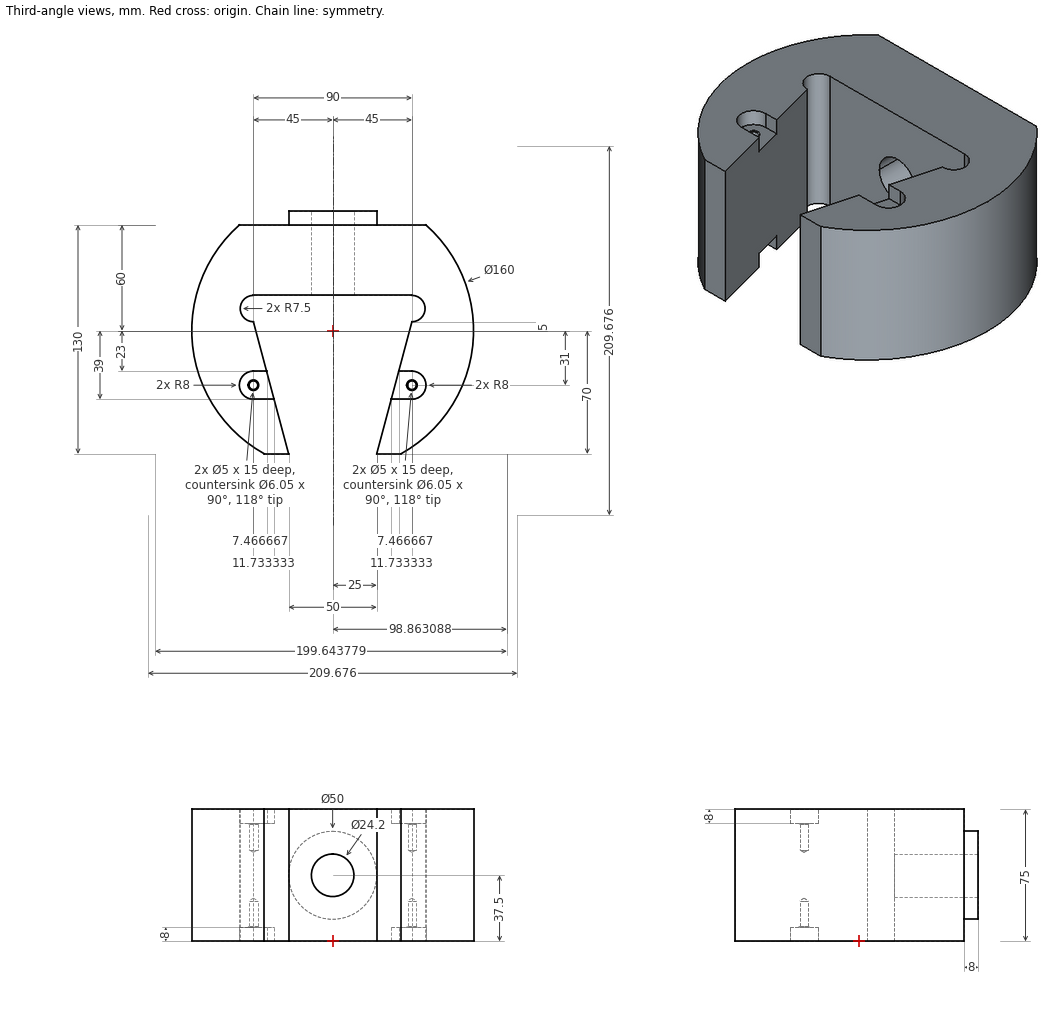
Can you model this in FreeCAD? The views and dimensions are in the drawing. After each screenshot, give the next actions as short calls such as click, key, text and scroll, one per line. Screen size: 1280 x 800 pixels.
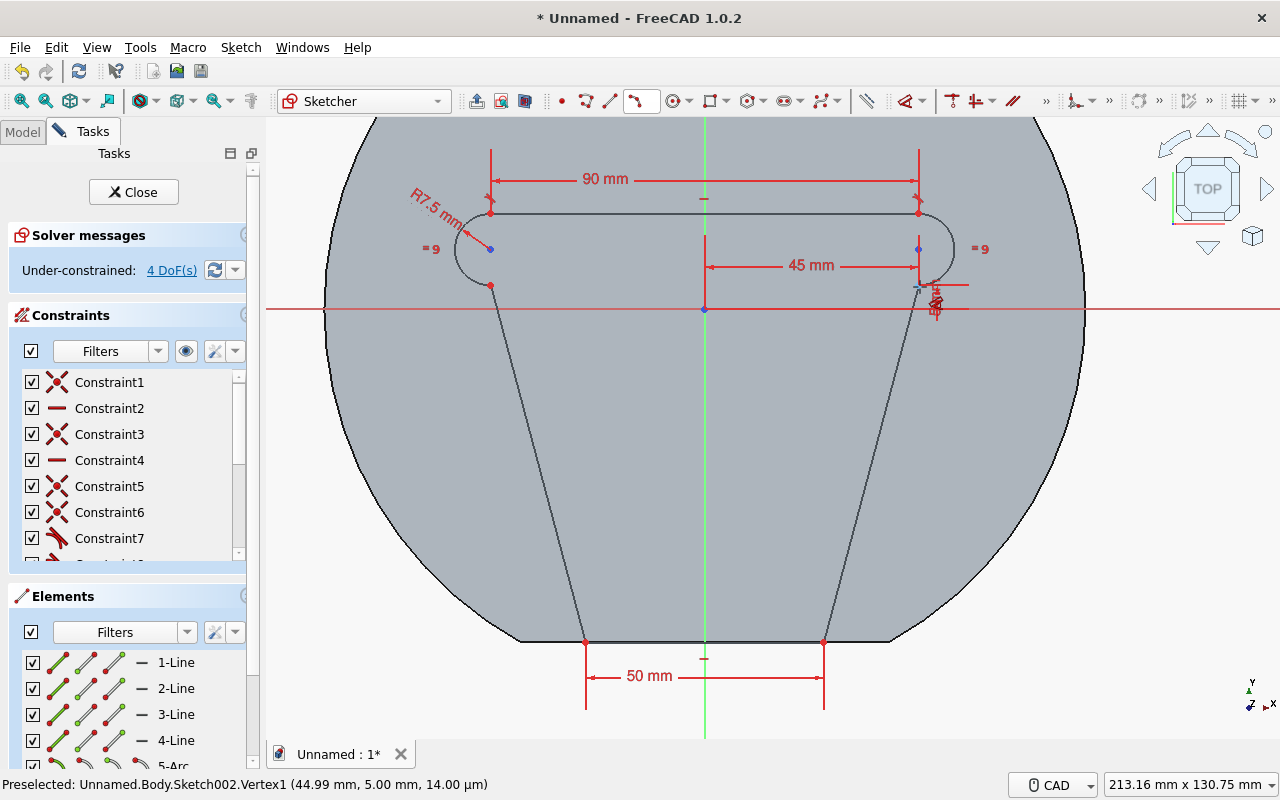
click(824, 643)
click(764, 677)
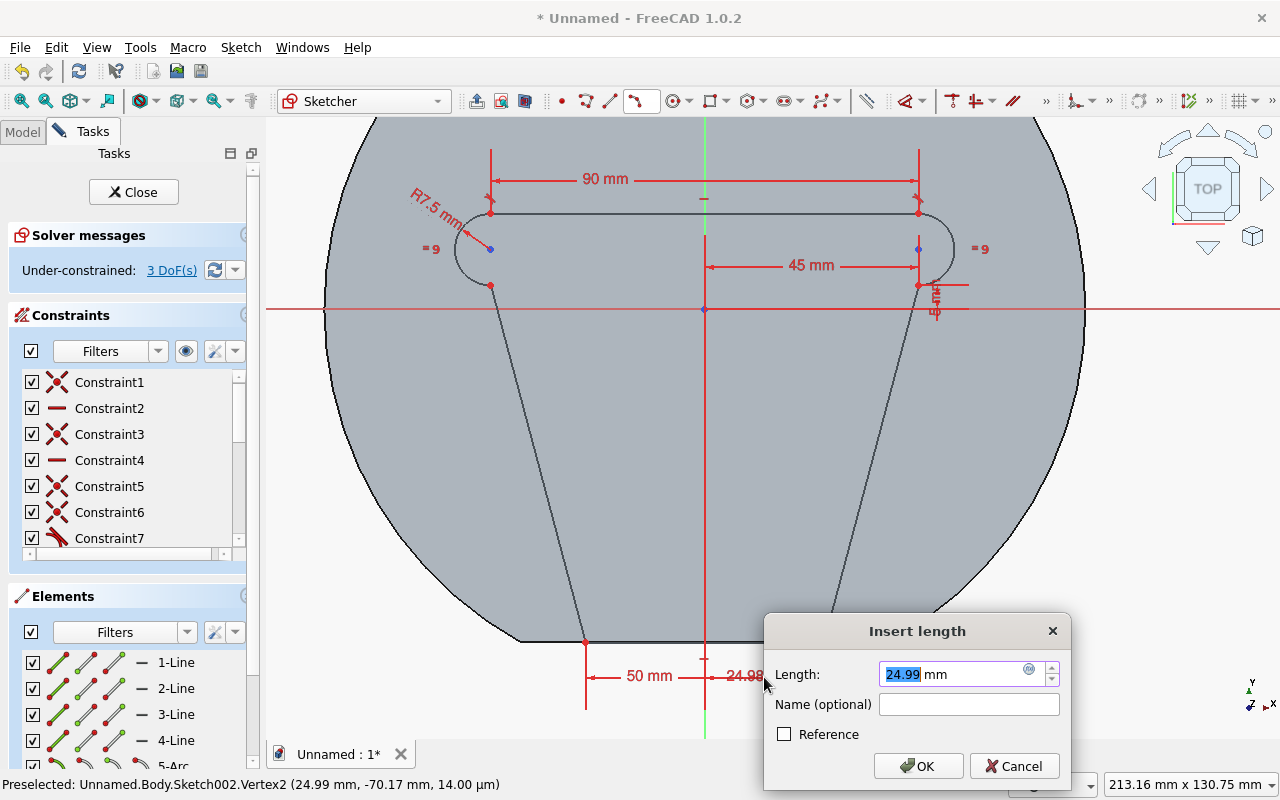
text(25)
key(Return)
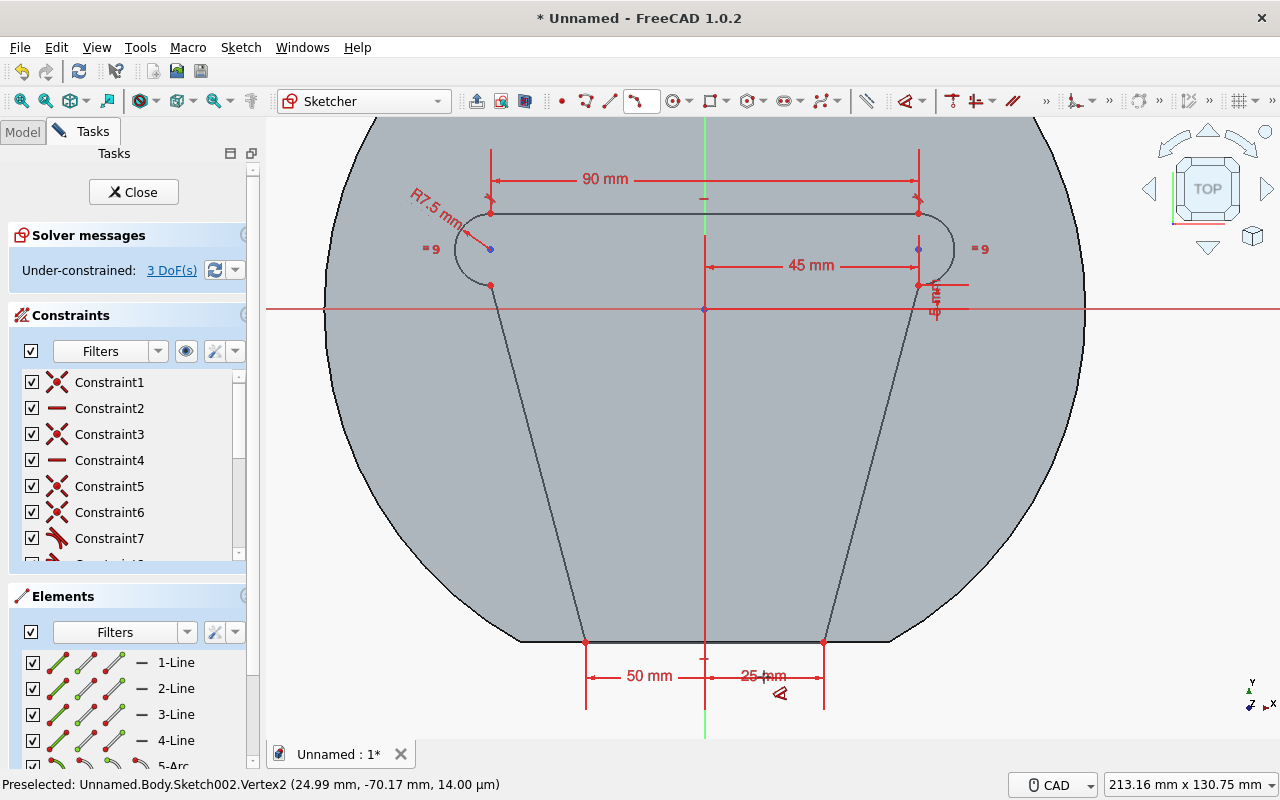
click(824, 643)
click(858, 399)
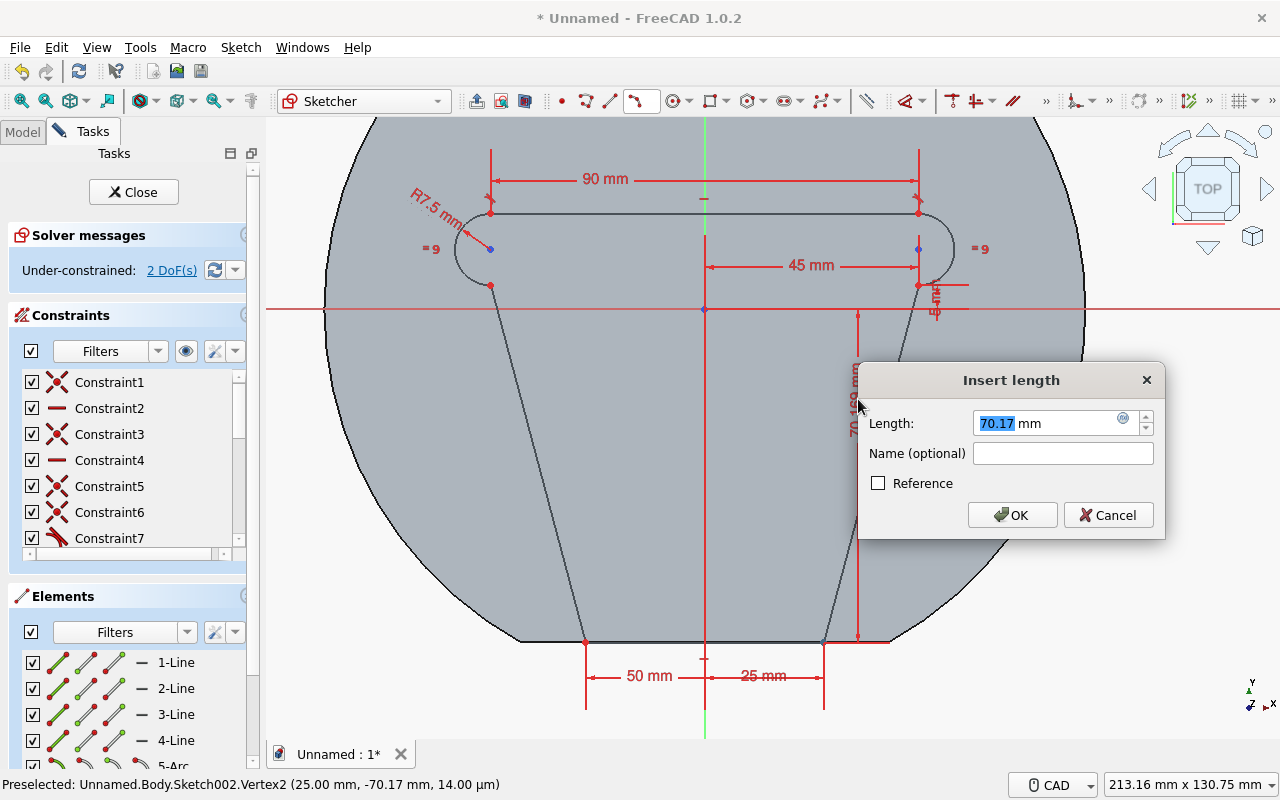
text(70)
key(Return)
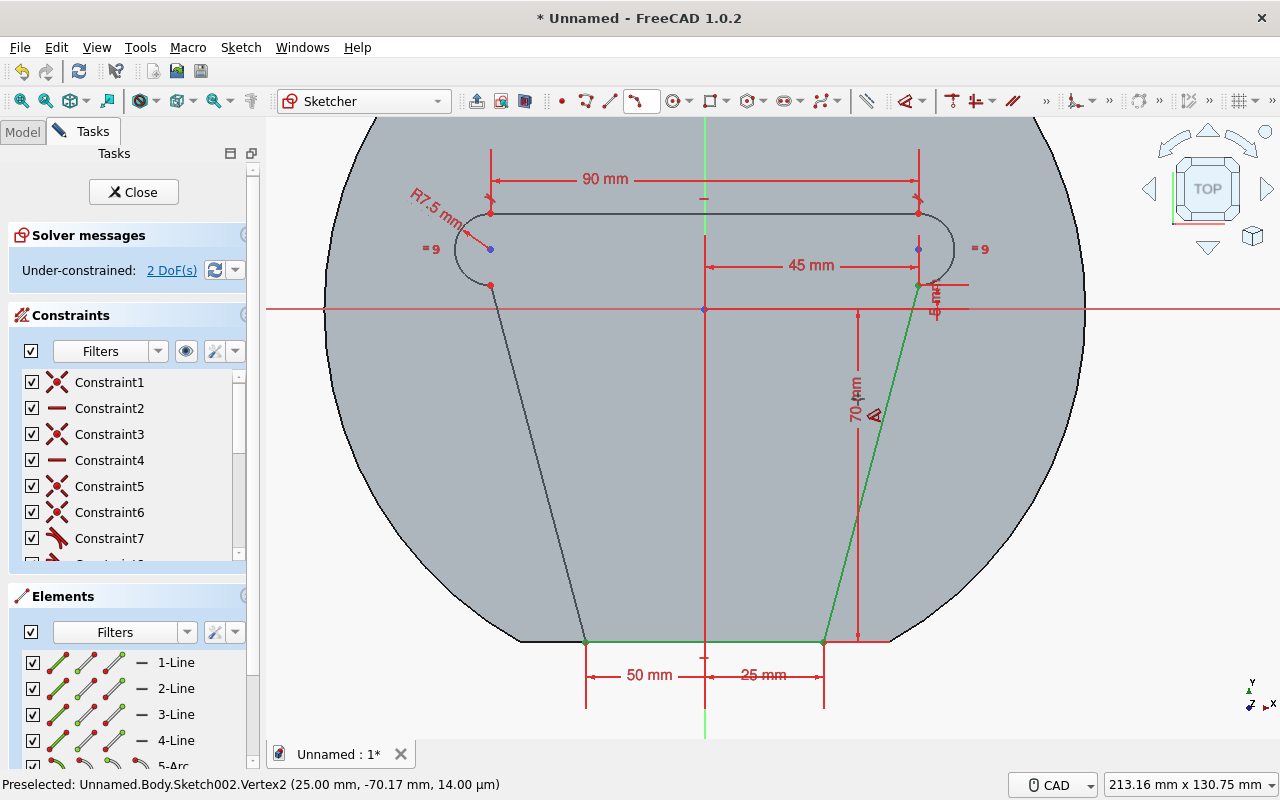
click(491, 285)
click(598, 251)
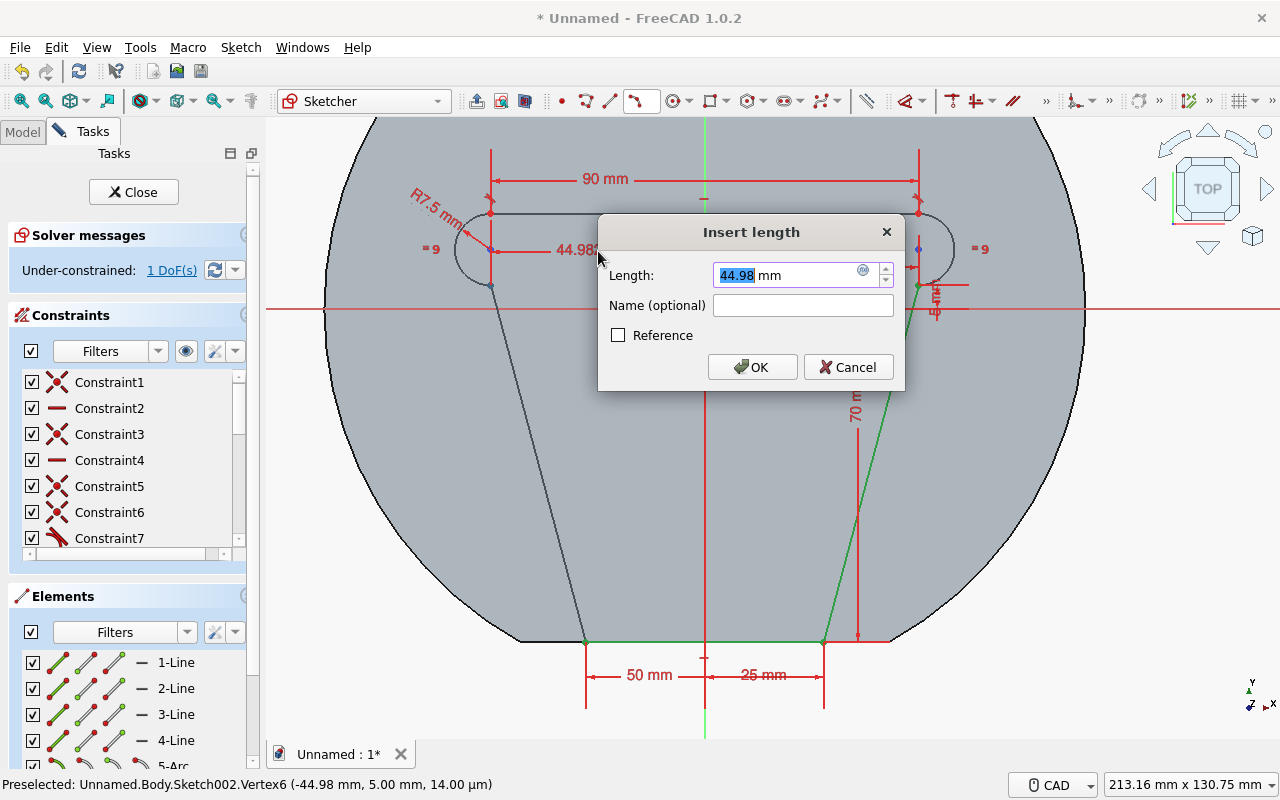
text(45)
key(Return)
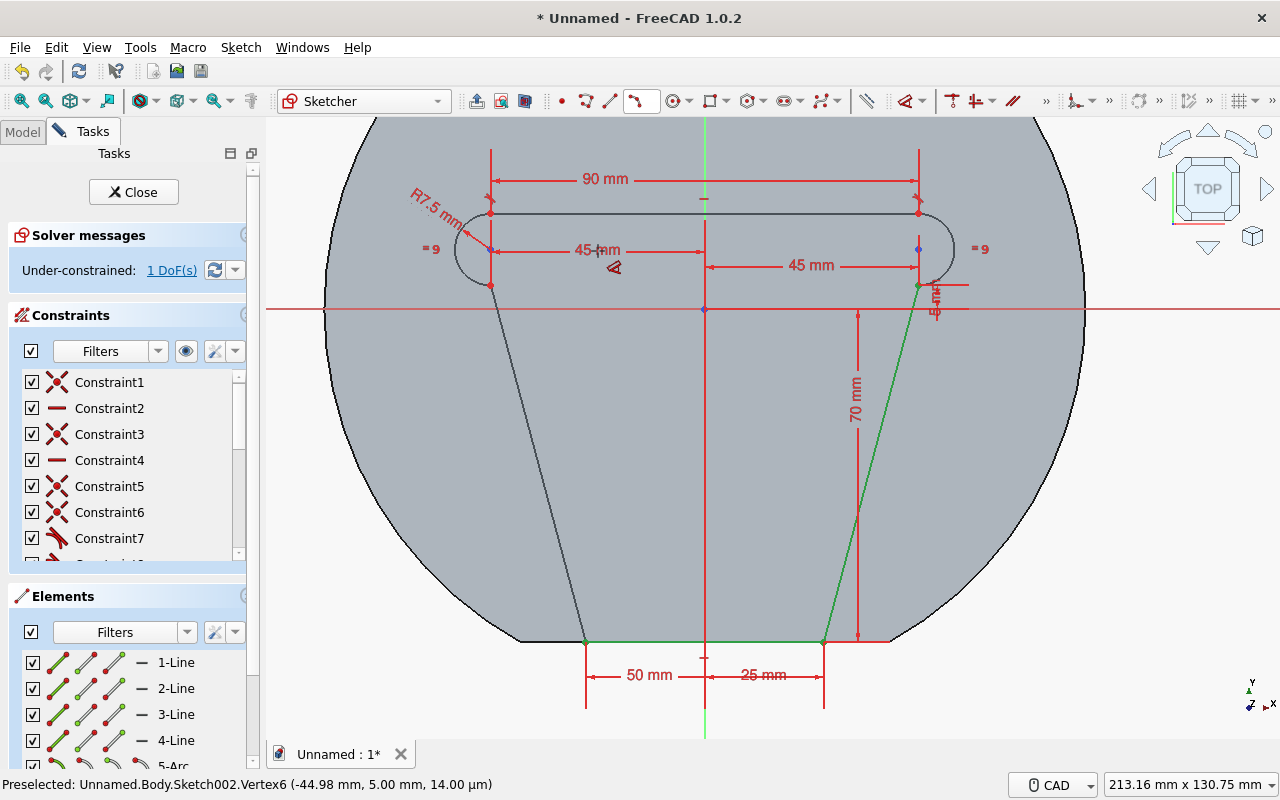
click(491, 214)
click(523, 180)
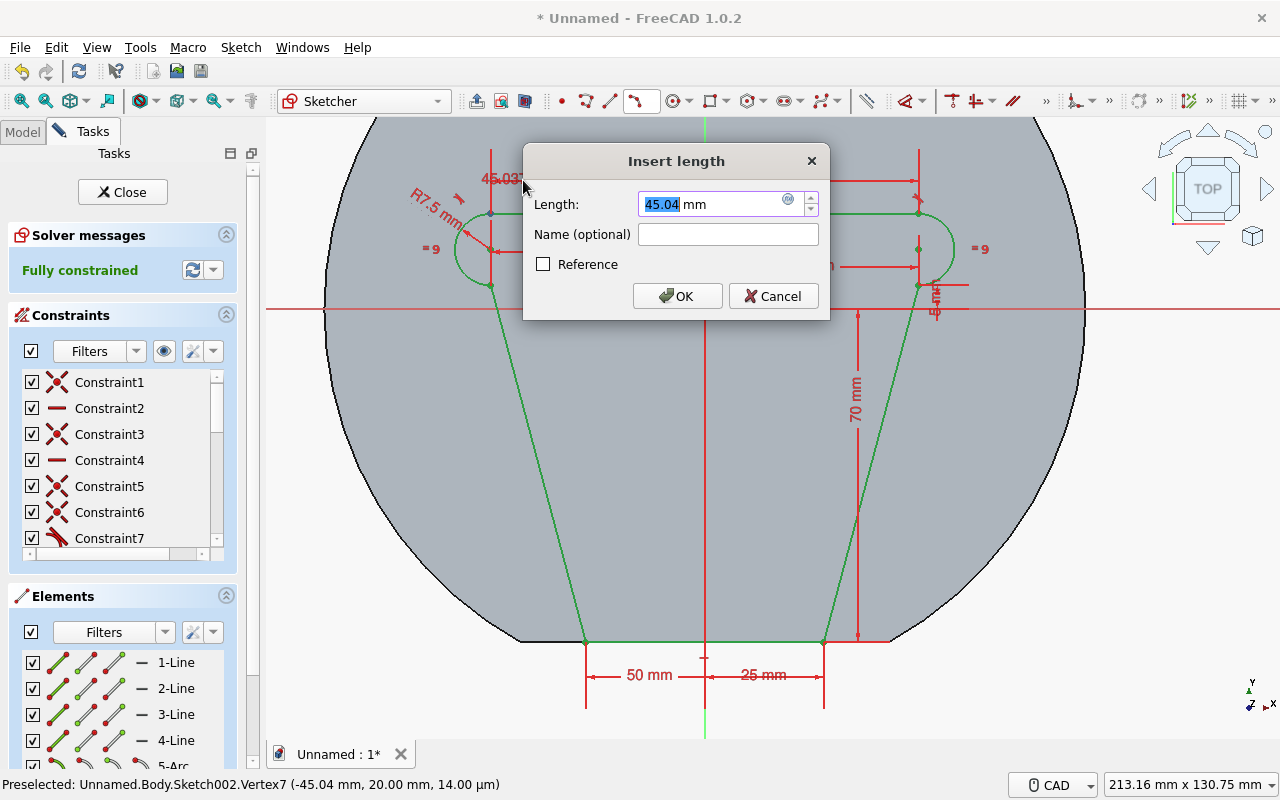
text(45)
key(Return)
key(Escape)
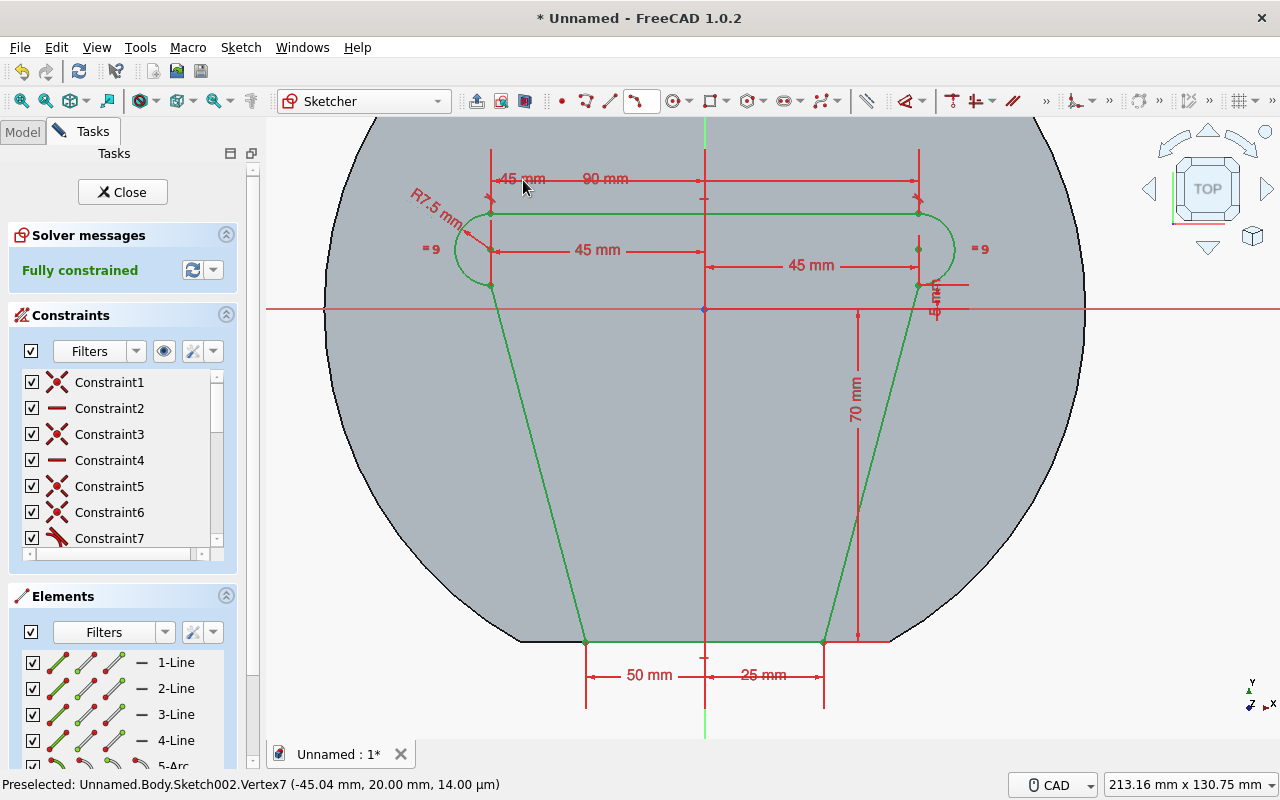
click(123, 192)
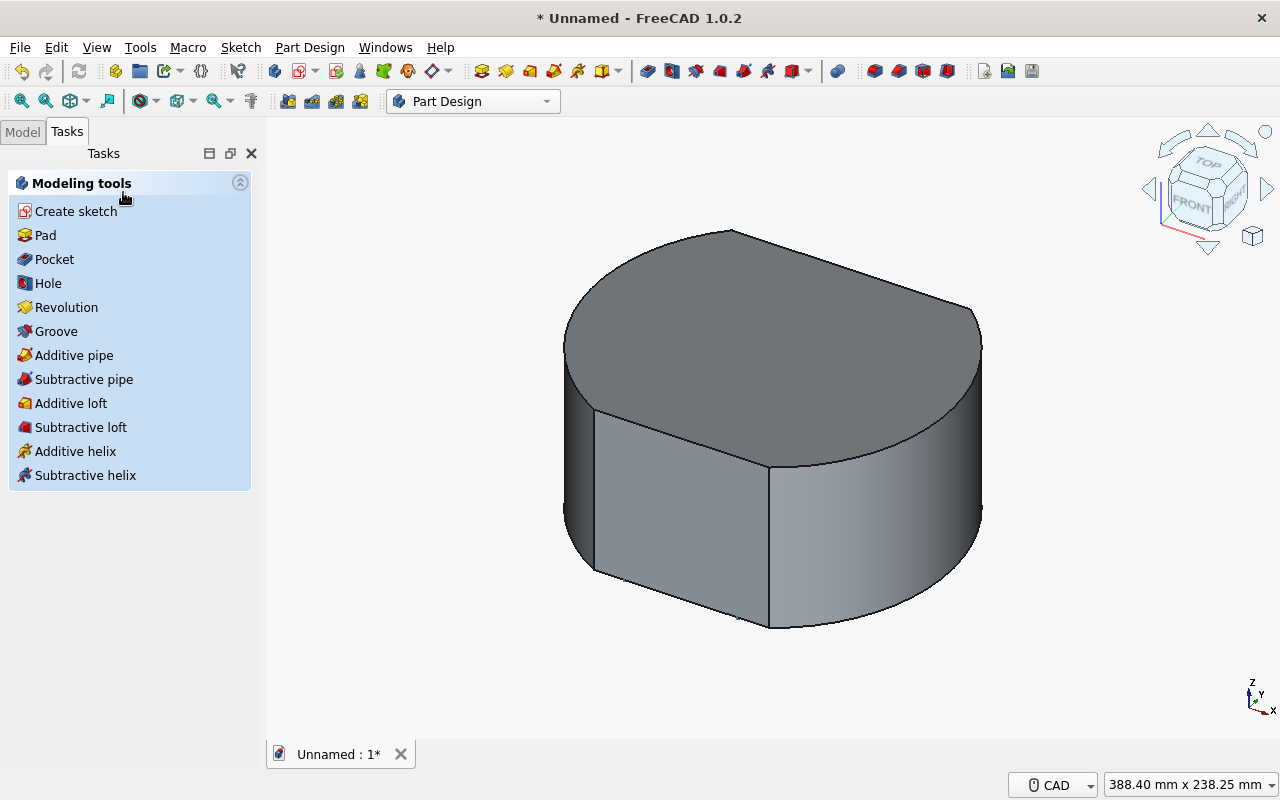
click(648, 72)